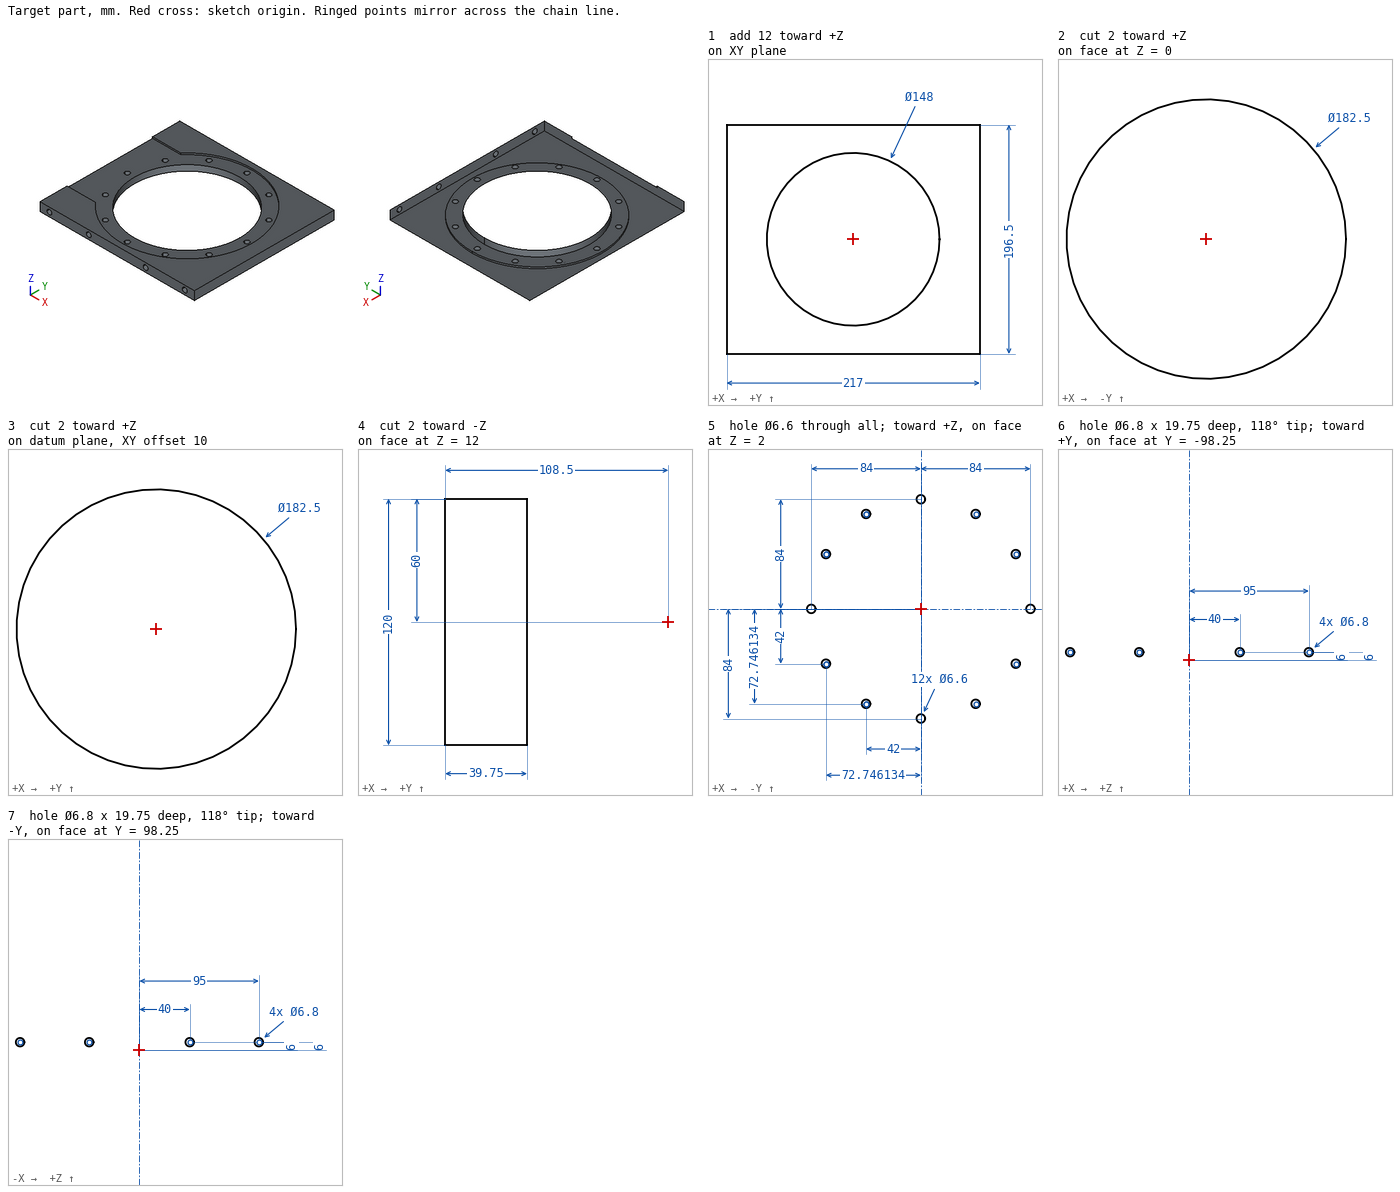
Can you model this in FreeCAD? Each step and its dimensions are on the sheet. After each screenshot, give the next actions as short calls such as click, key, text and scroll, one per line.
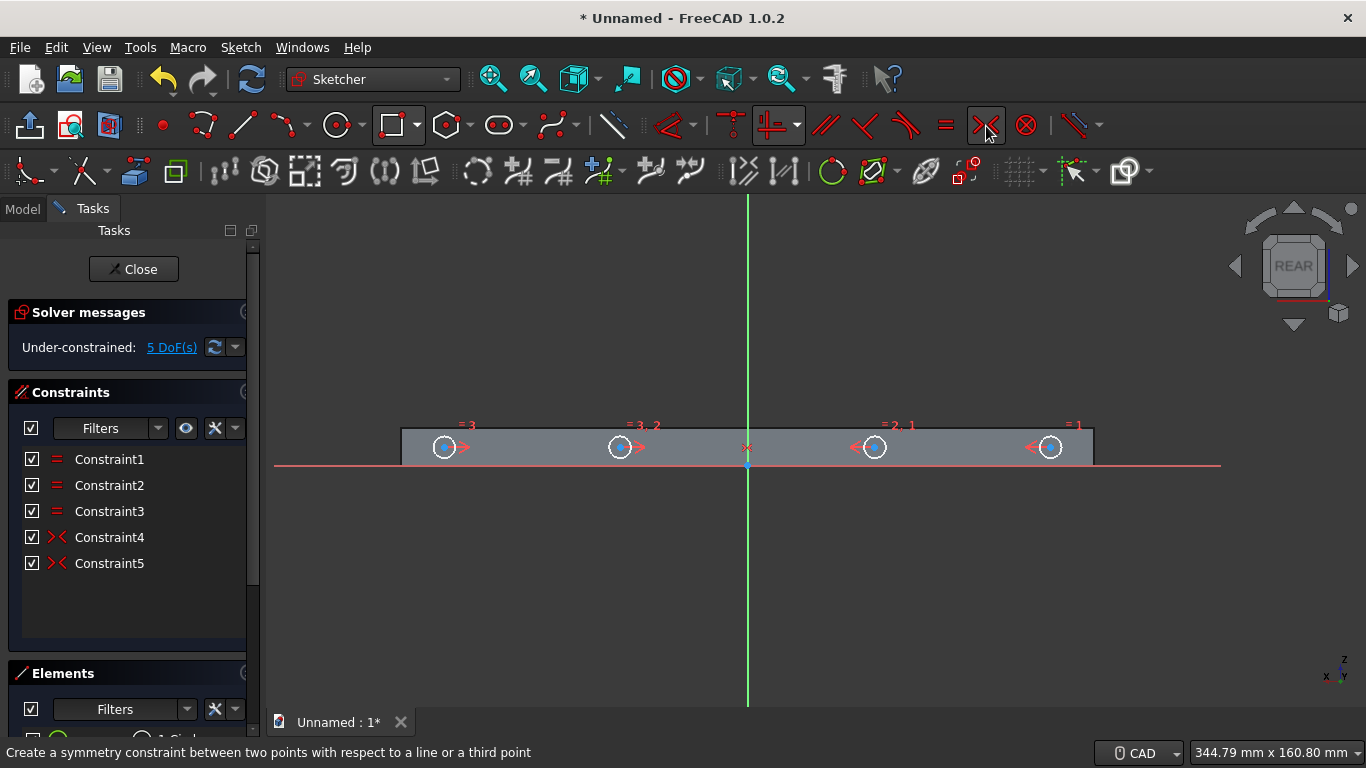
click(668, 126)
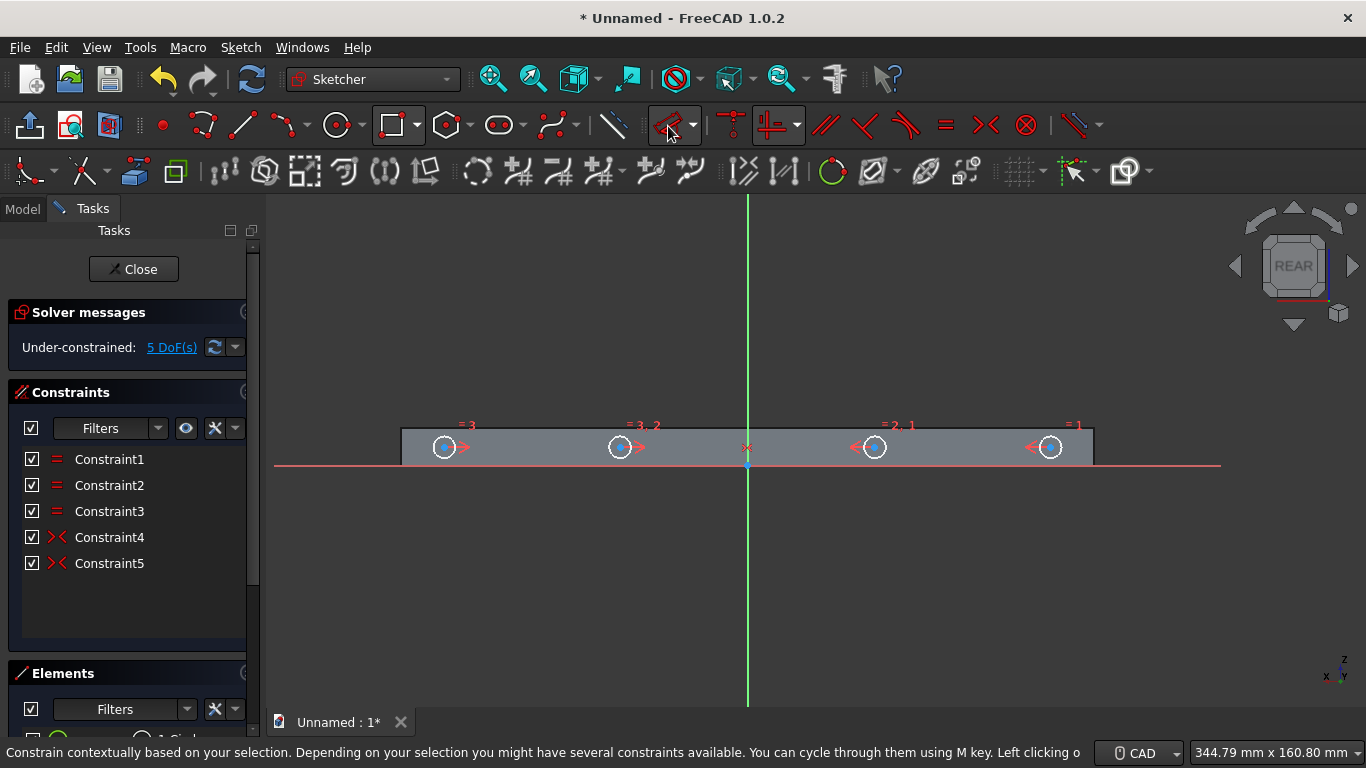
scroll(1058, 440, up, 4)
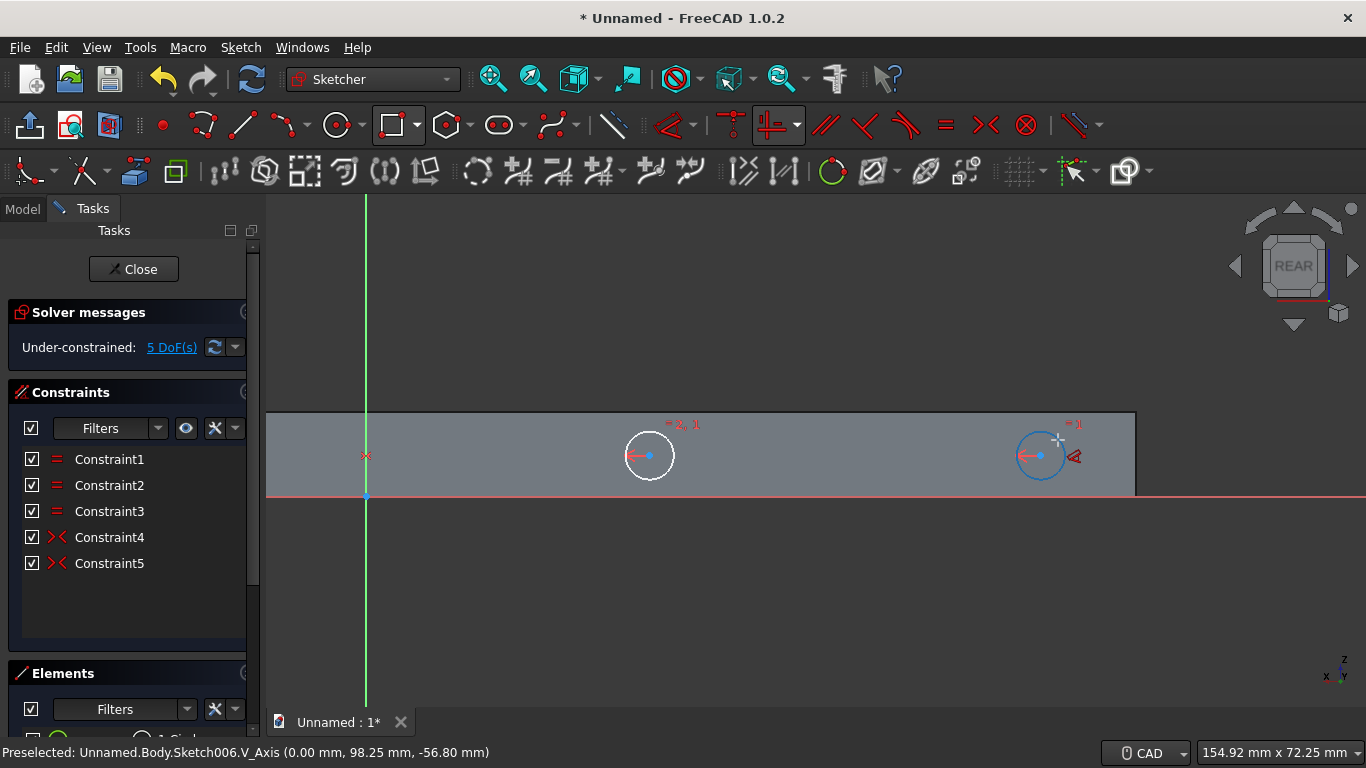
click(1058, 439)
click(1081, 417)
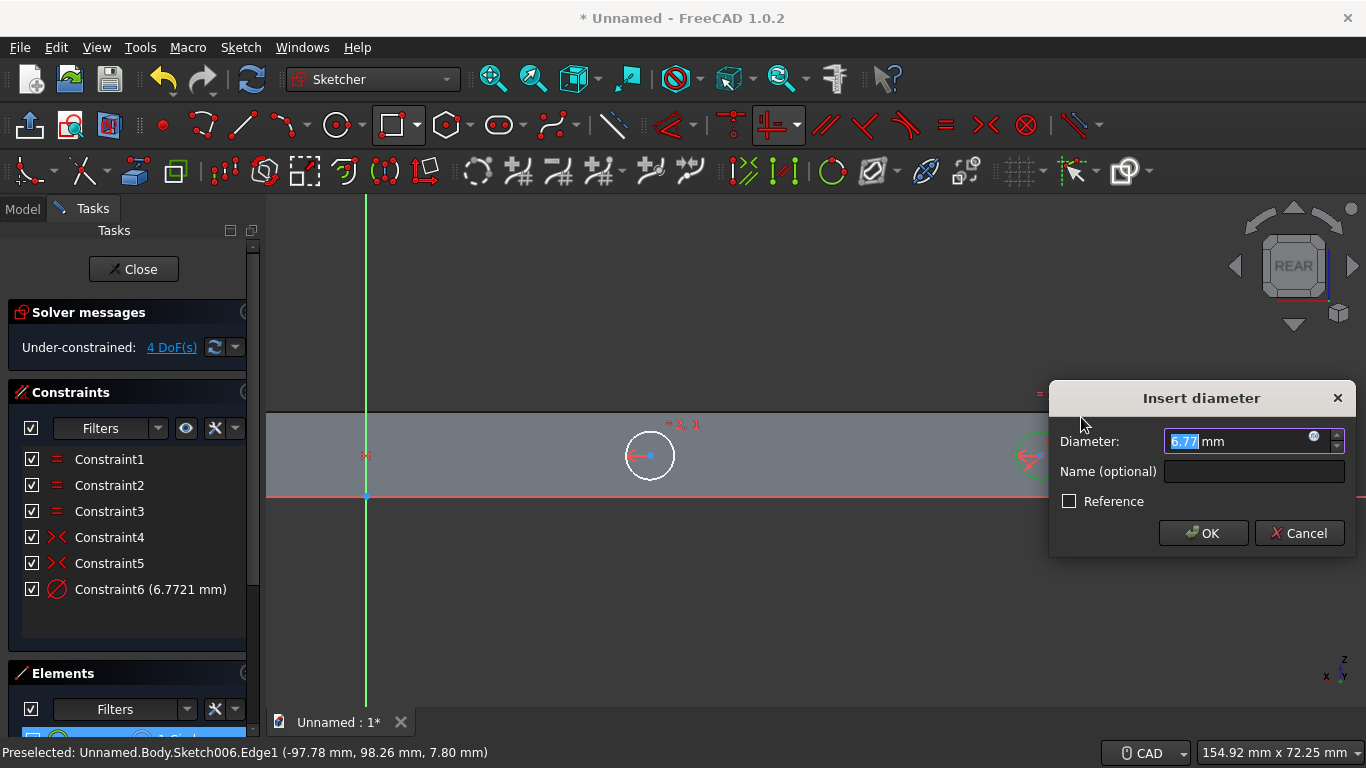
text(6.8)
key(Return)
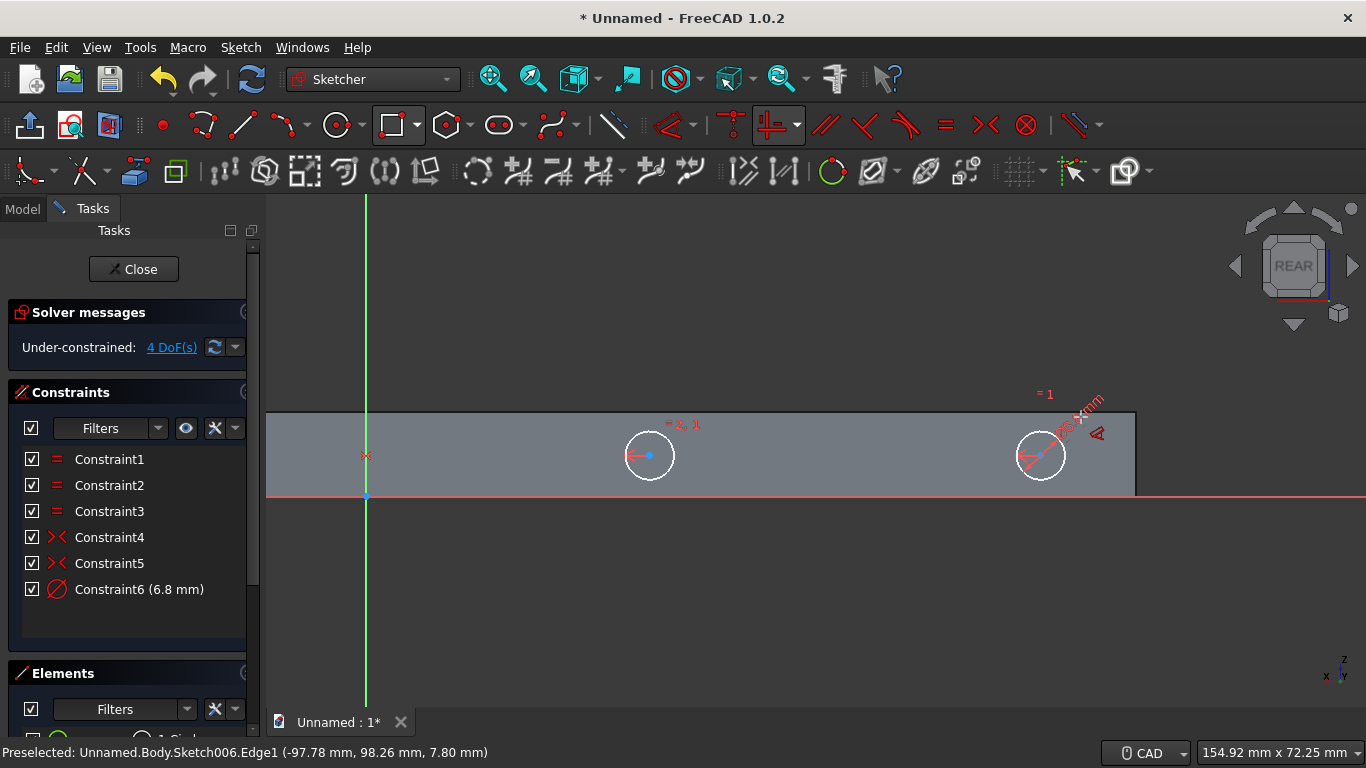
click(1041, 456)
click(1075, 476)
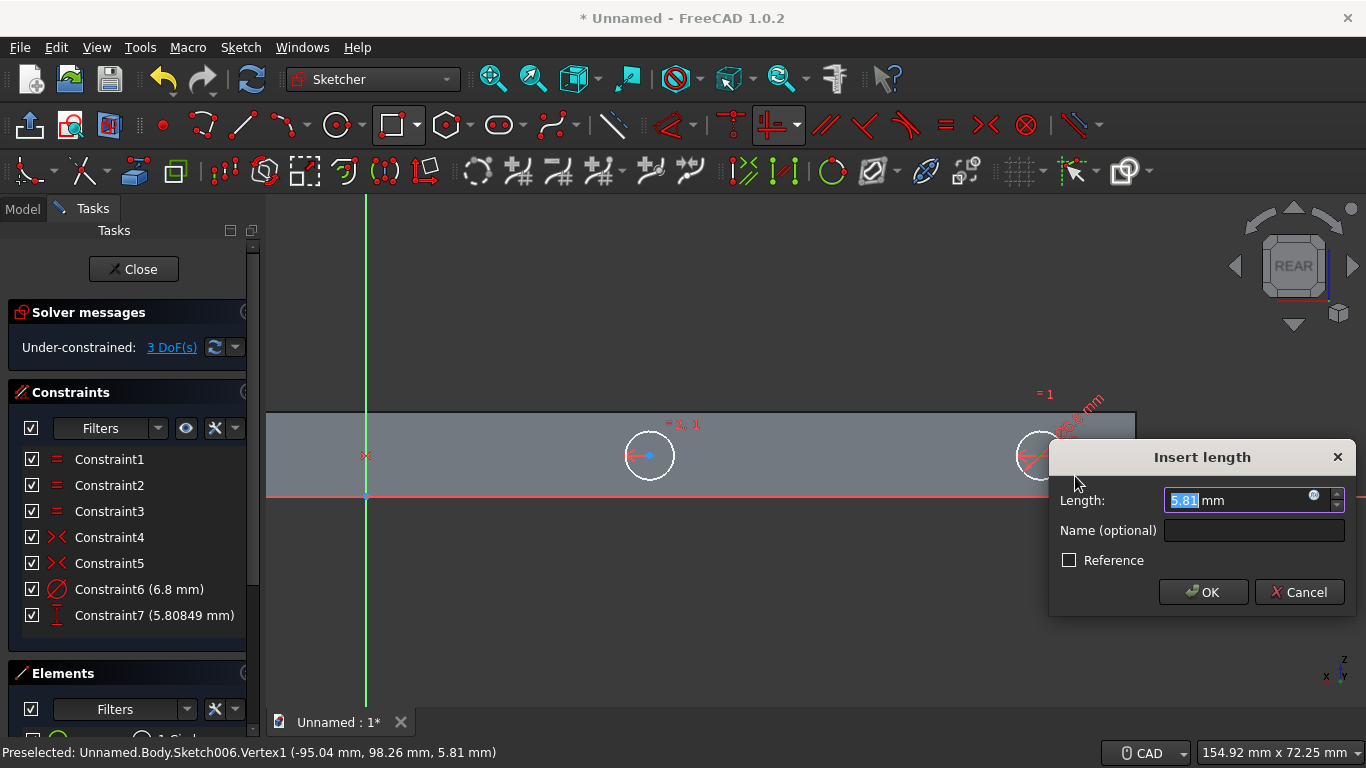
text(6)
key(Return)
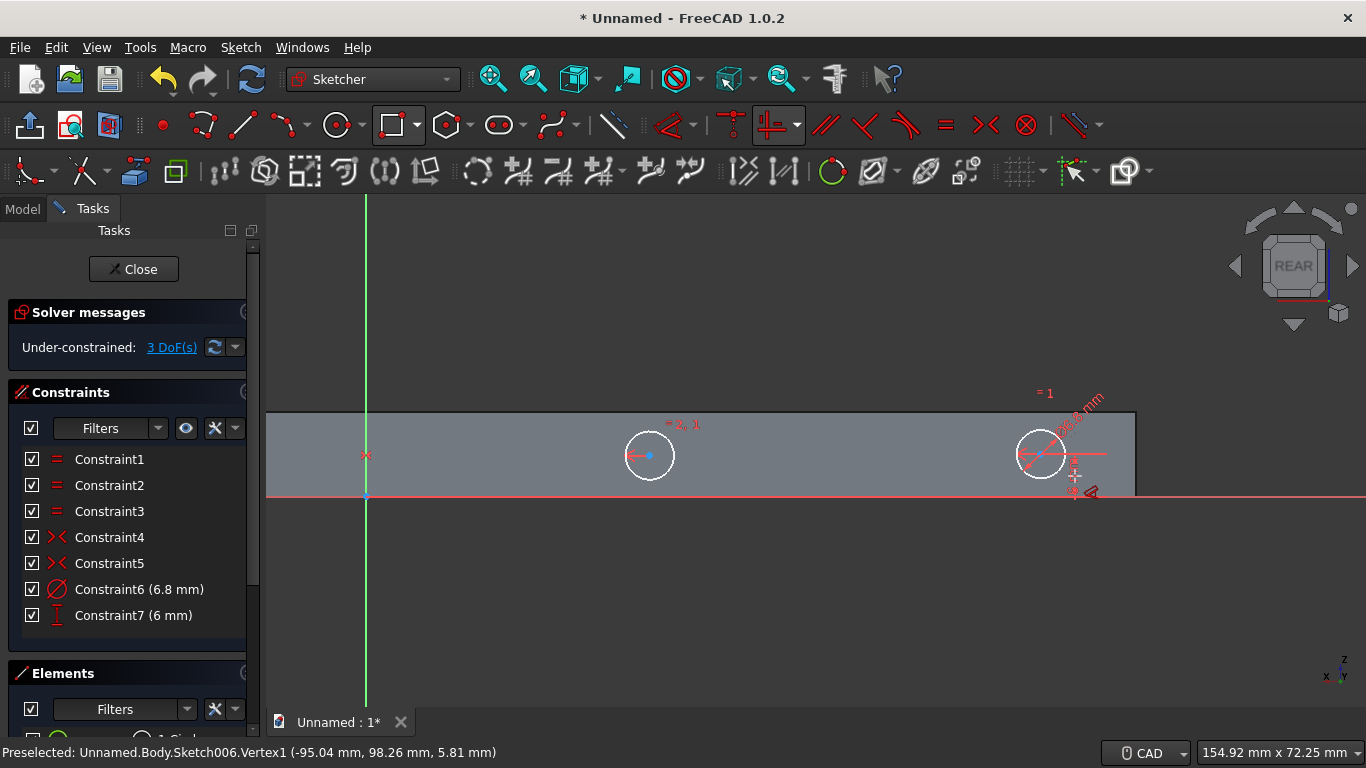
click(650, 456)
click(684, 476)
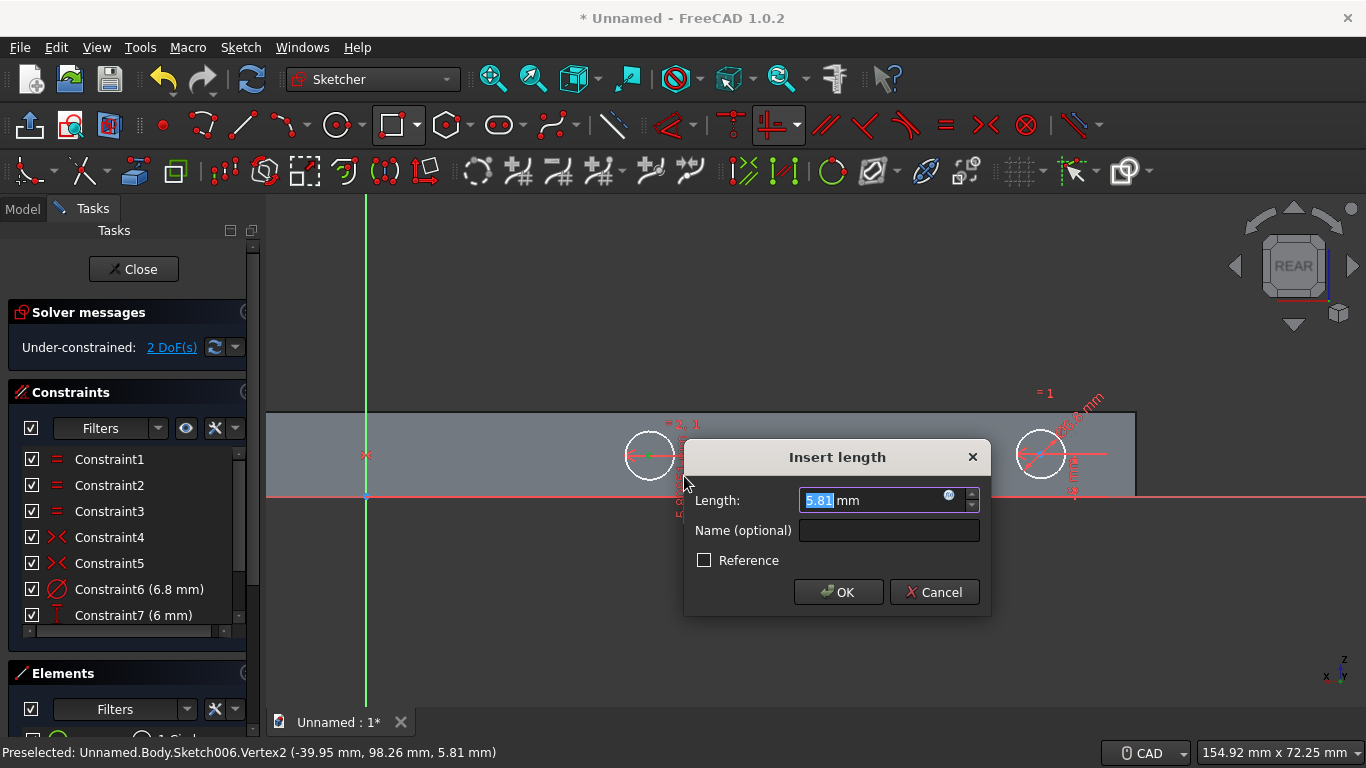
text(6)
key(Return)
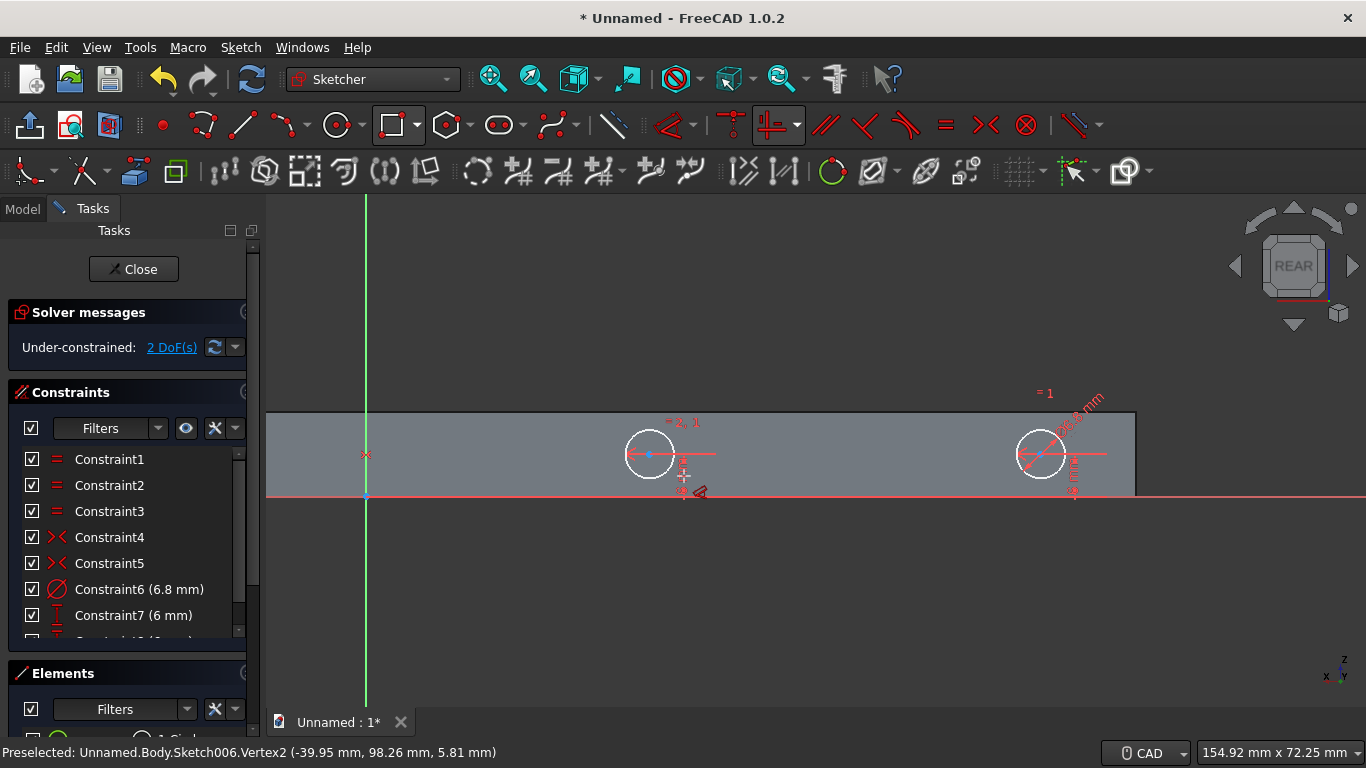
click(1041, 454)
click(703, 531)